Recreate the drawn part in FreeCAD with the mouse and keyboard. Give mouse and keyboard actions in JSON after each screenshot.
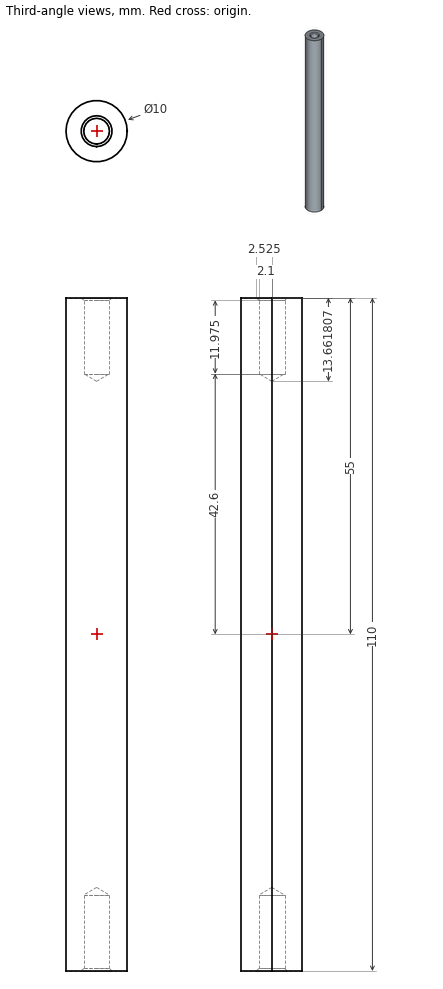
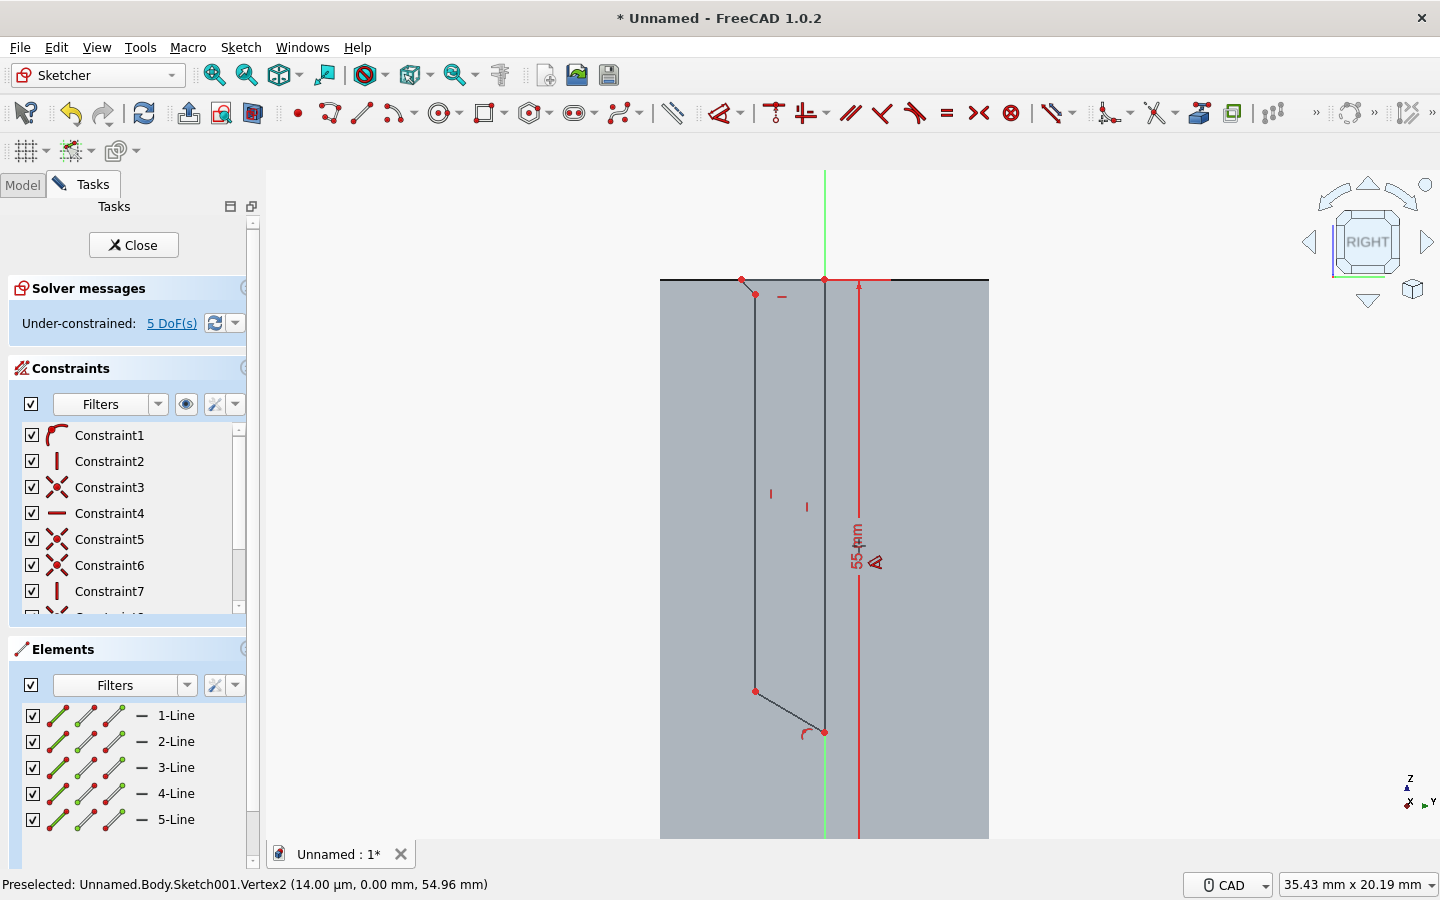
{"action": "left_click", "coordinate": [755, 295]}
{"action": "left_click", "coordinate": [790, 261]}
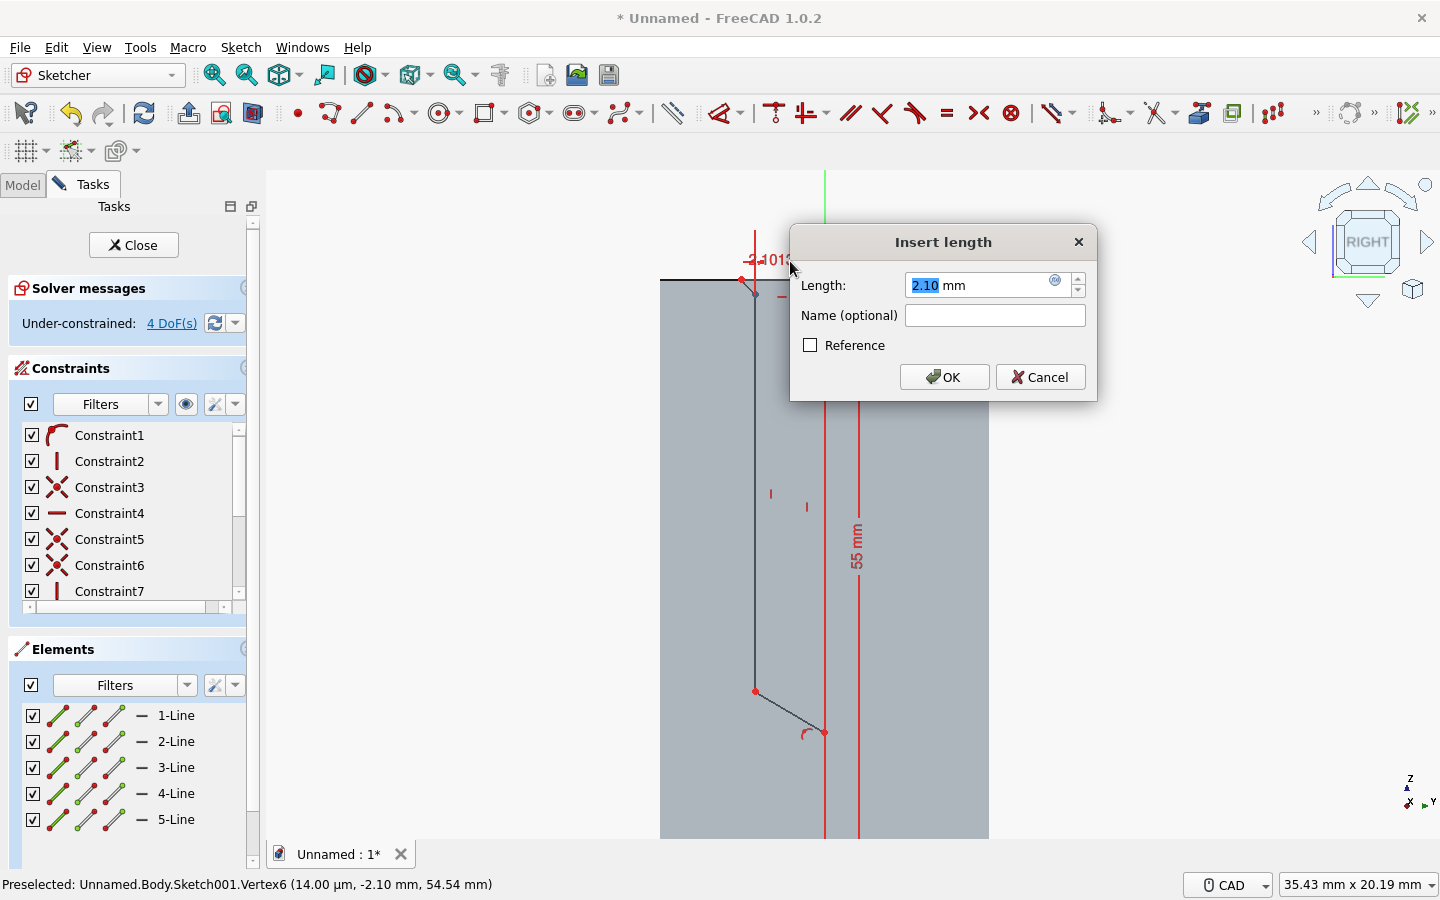
{"action": "type", "text": "2.1"}
{"action": "key", "text": "Return"}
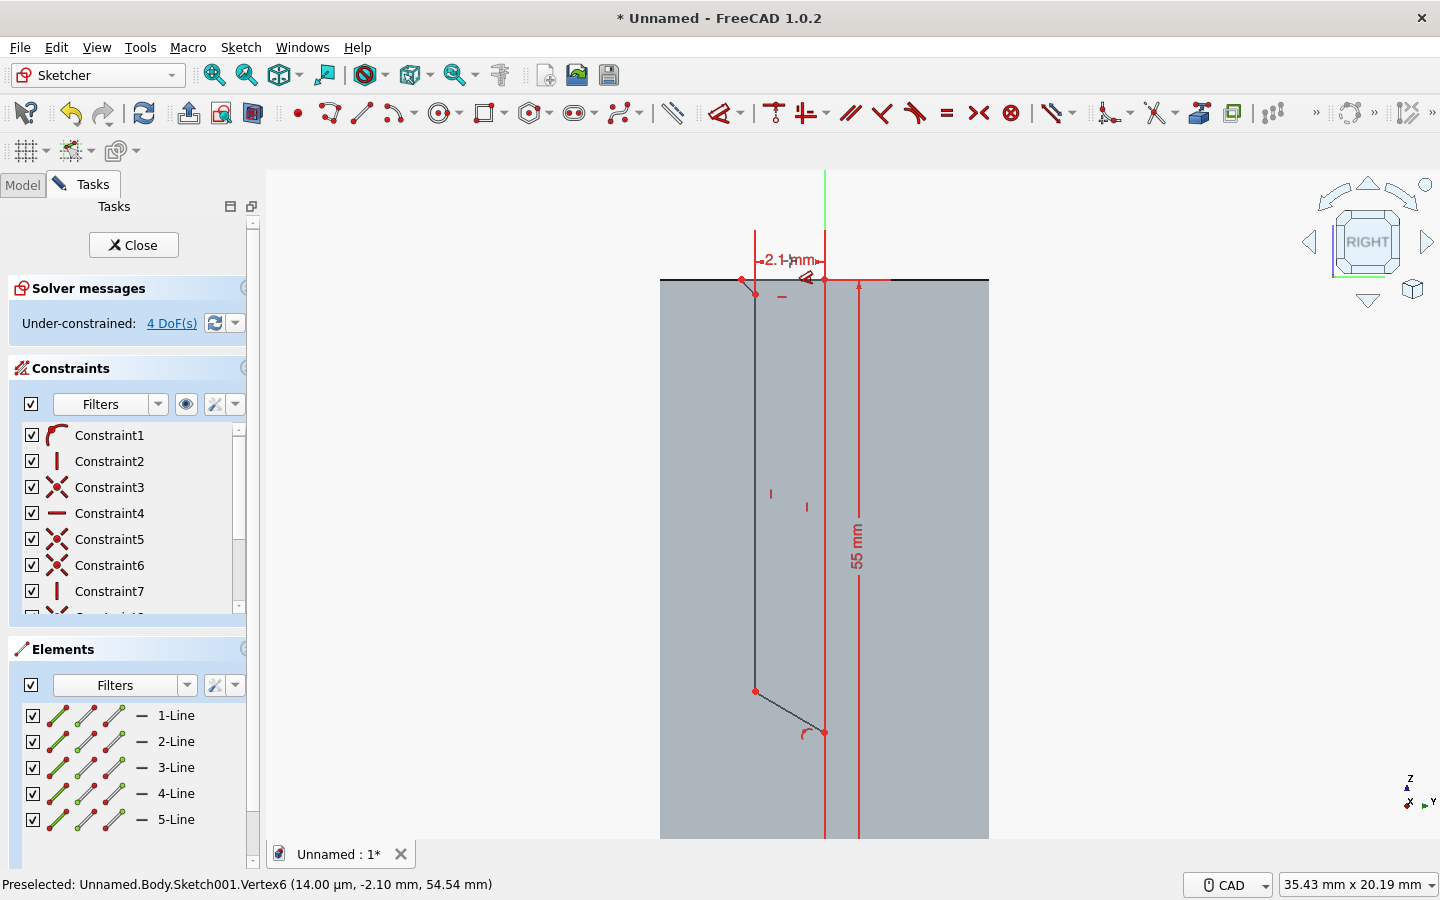
{"action": "left_click", "coordinate": [800, 280]}
{"action": "left_click", "coordinate": [783, 314]}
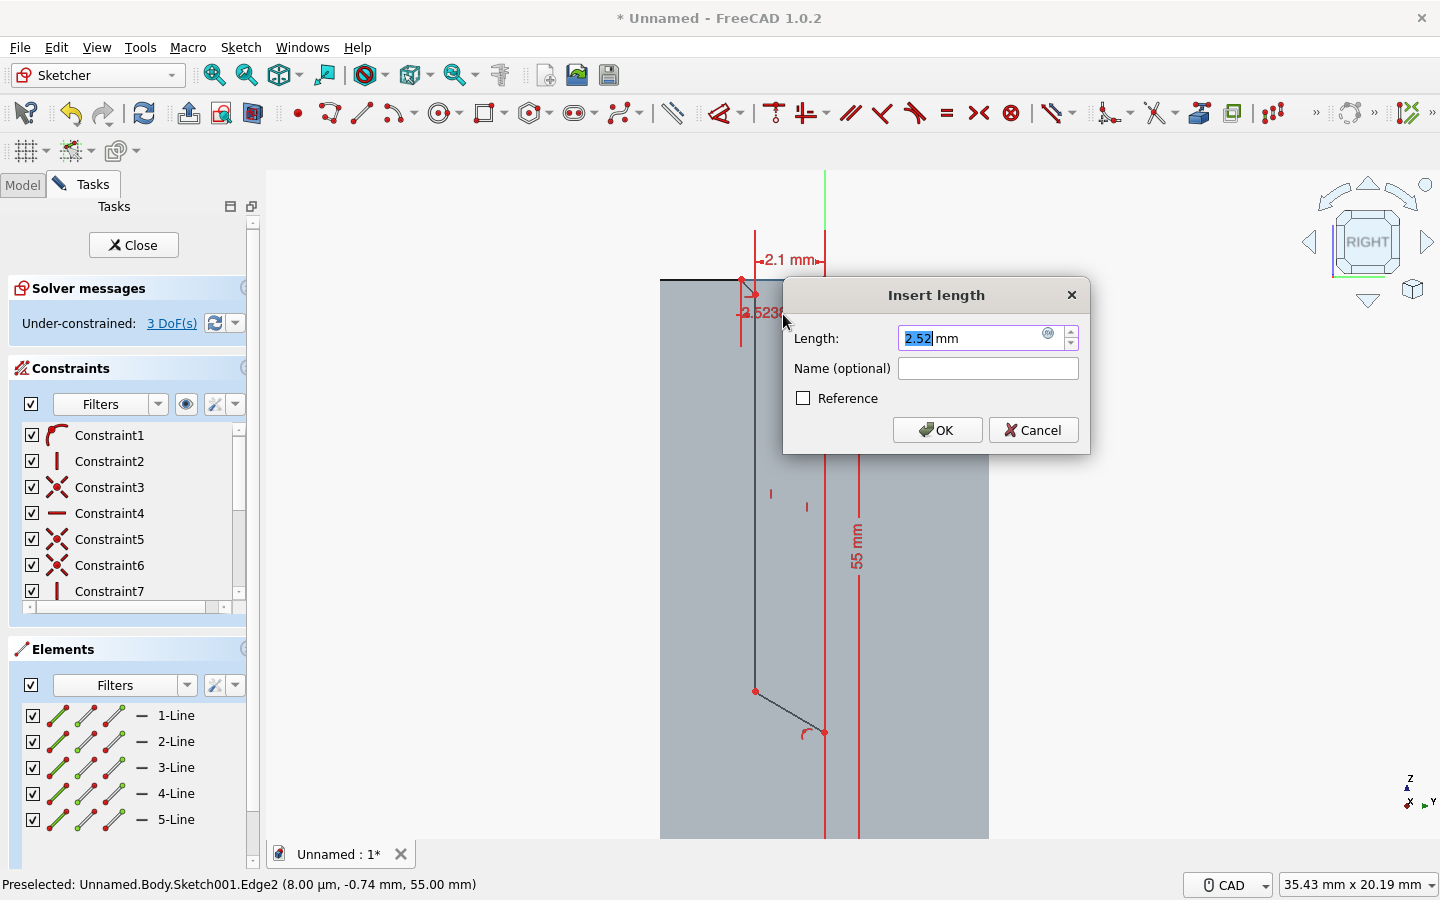
{"action": "type", "text": "2.525"}
{"action": "key", "text": "Return"}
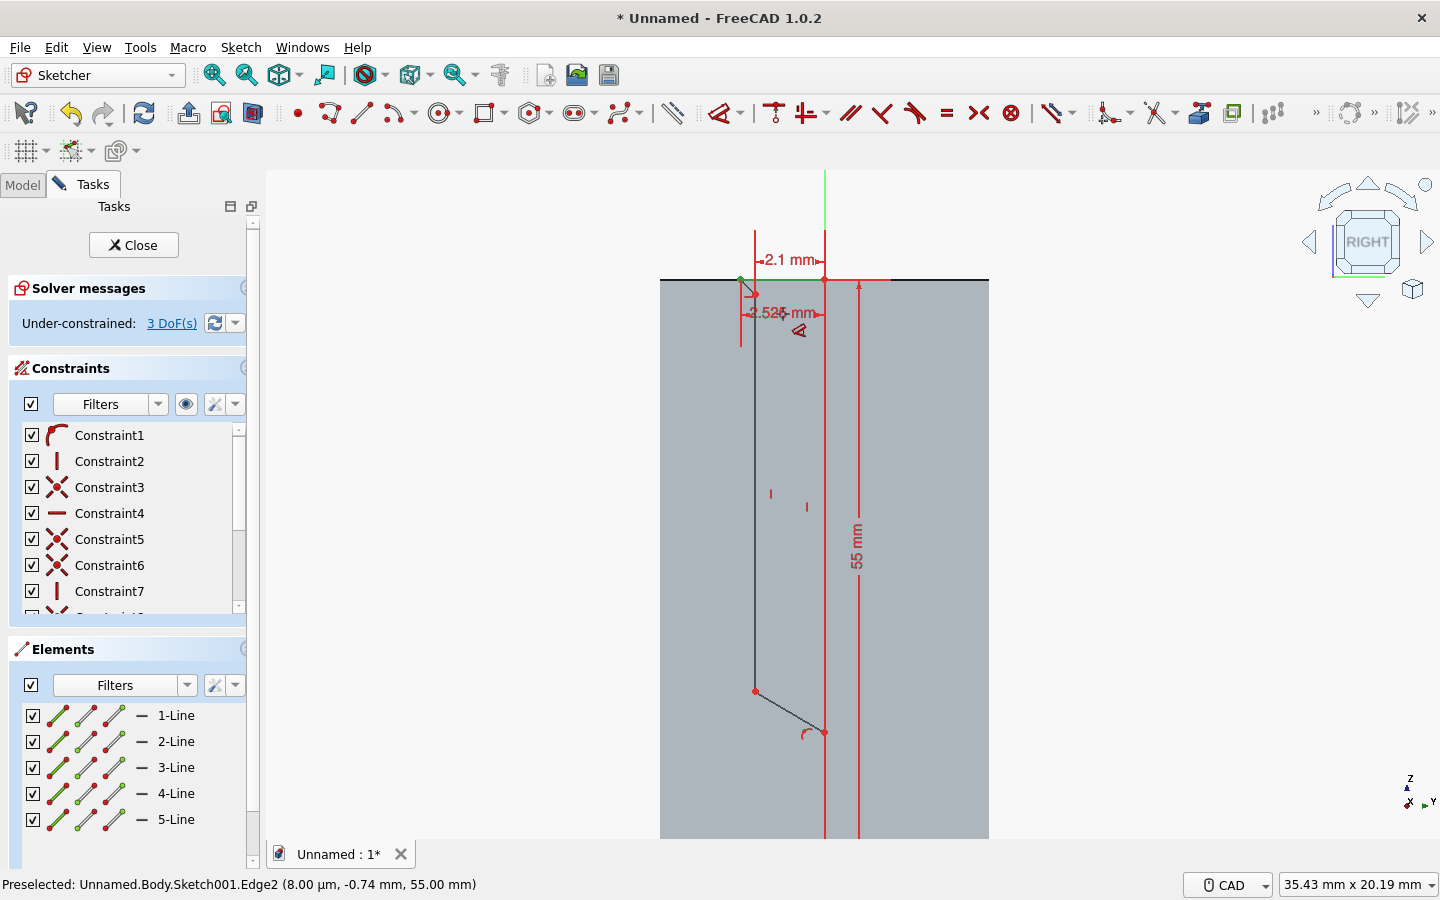
{"action": "left_click", "coordinate": [755, 692]}
{"action": "left_click", "coordinate": [859, 751]}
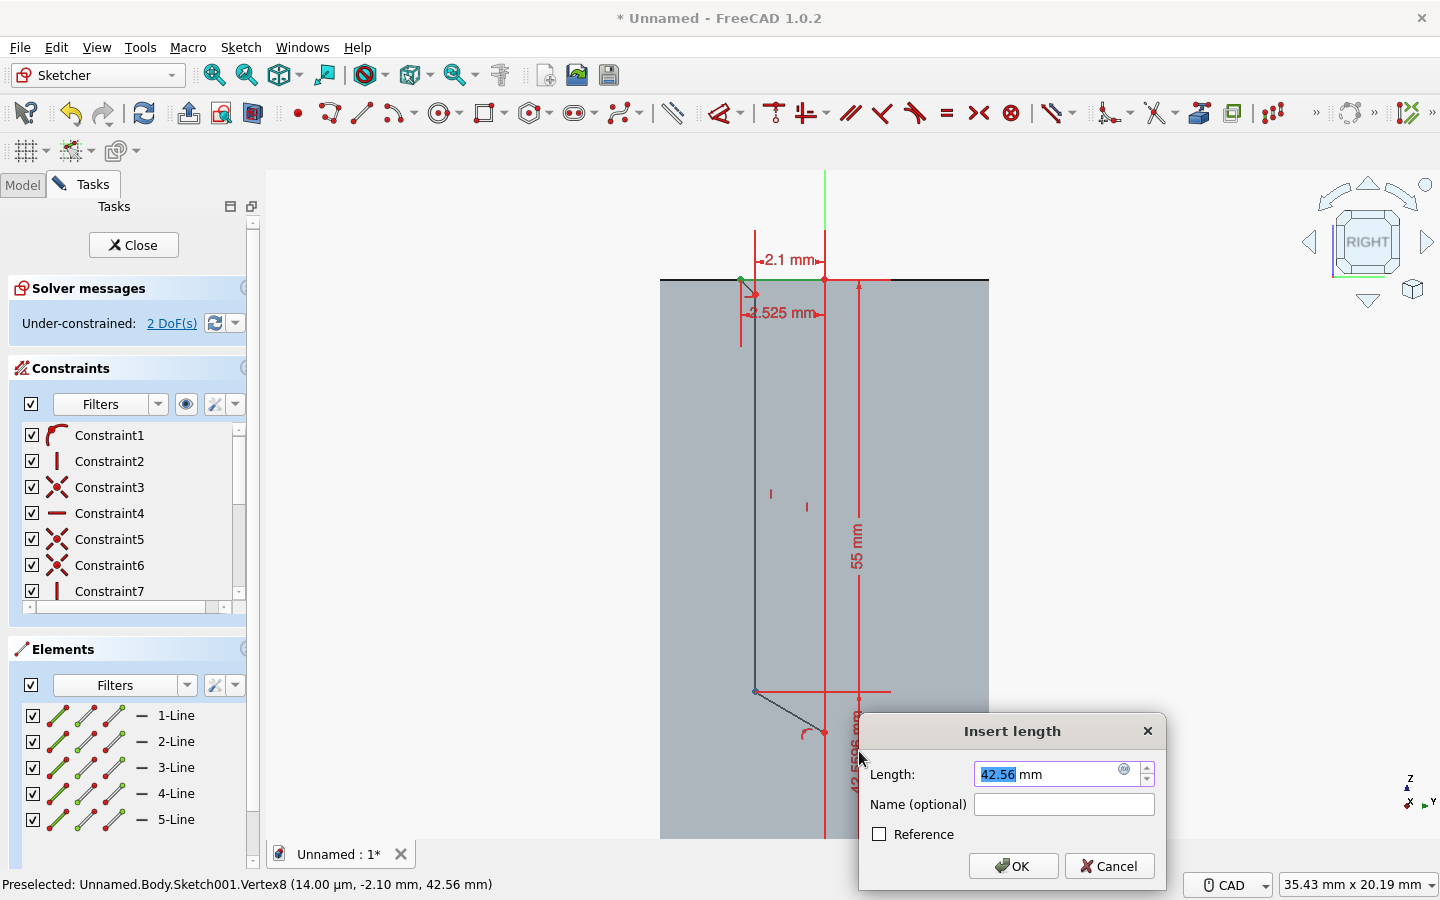
{"action": "type", "text": "42.6"}
{"action": "key", "text": "Return"}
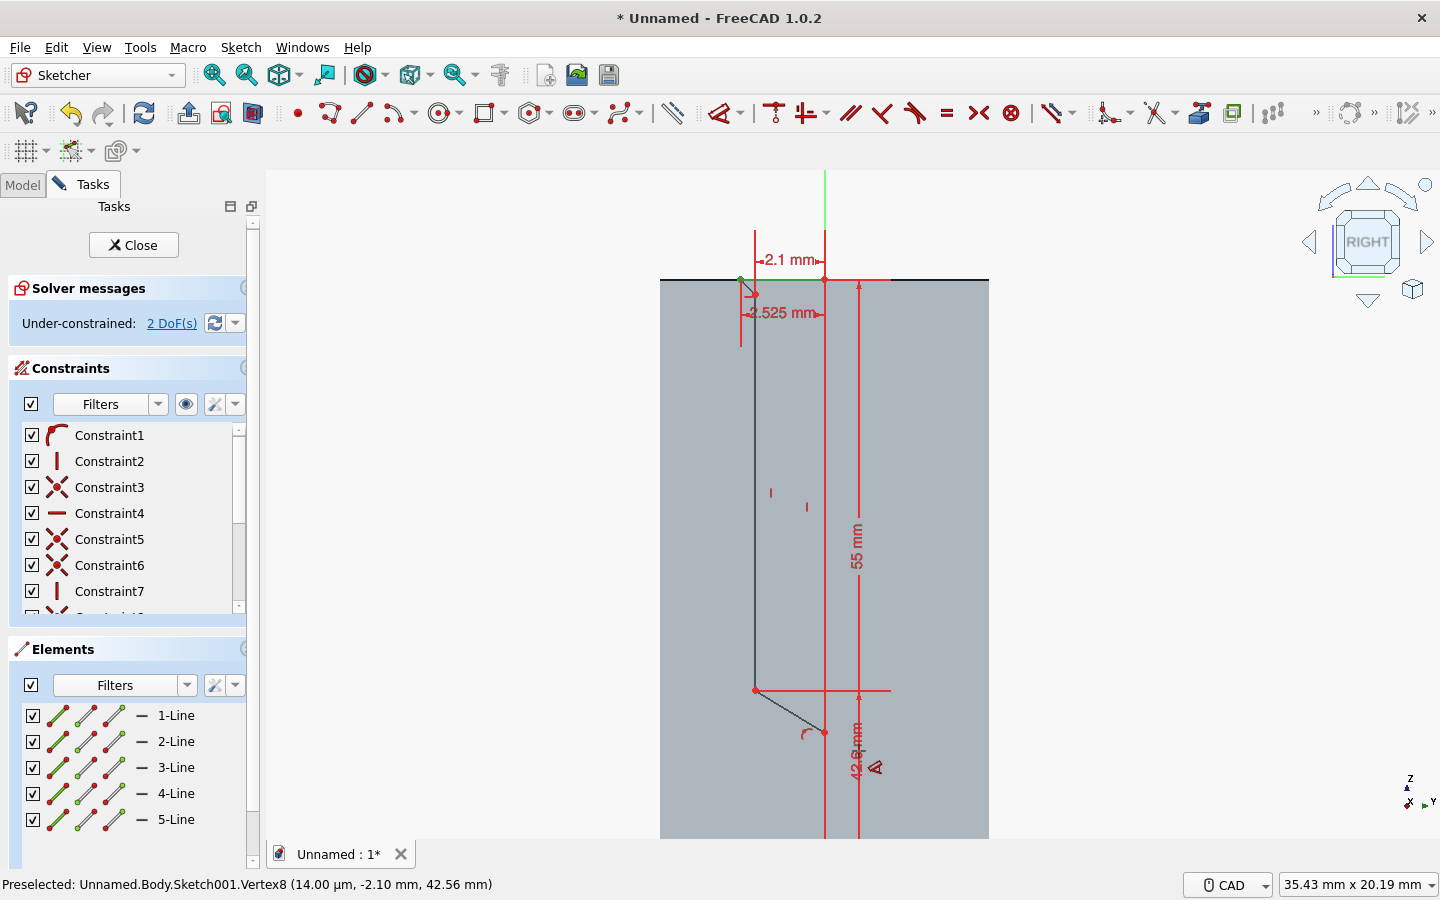
{"action": "left_click", "coordinate": [755, 414]}
{"action": "left_click", "coordinate": [721, 493]}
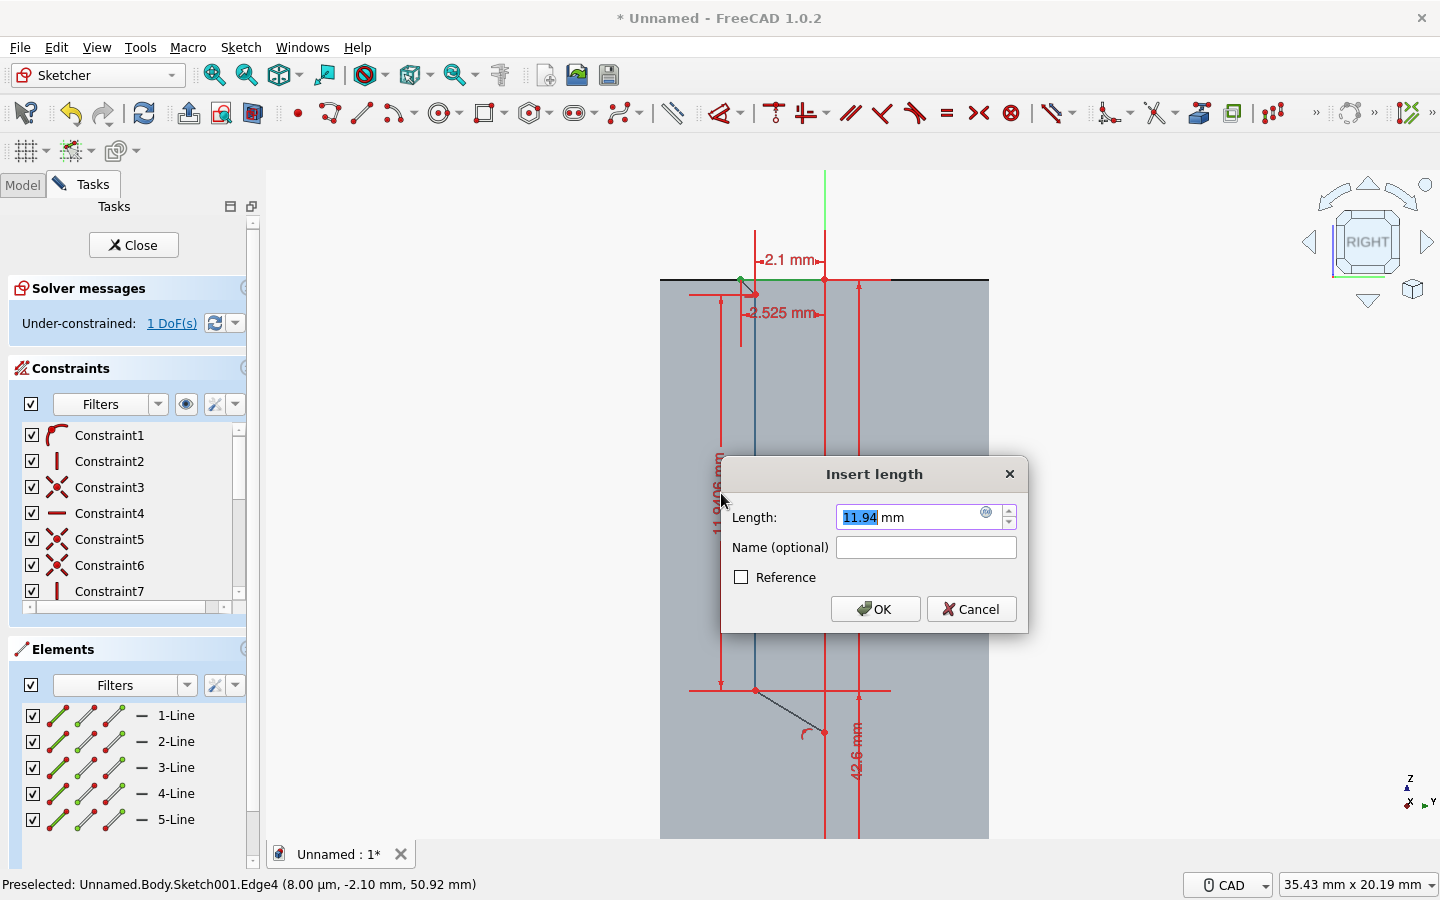
{"action": "type", "text": "11.975"}
{"action": "key", "text": "Return"}